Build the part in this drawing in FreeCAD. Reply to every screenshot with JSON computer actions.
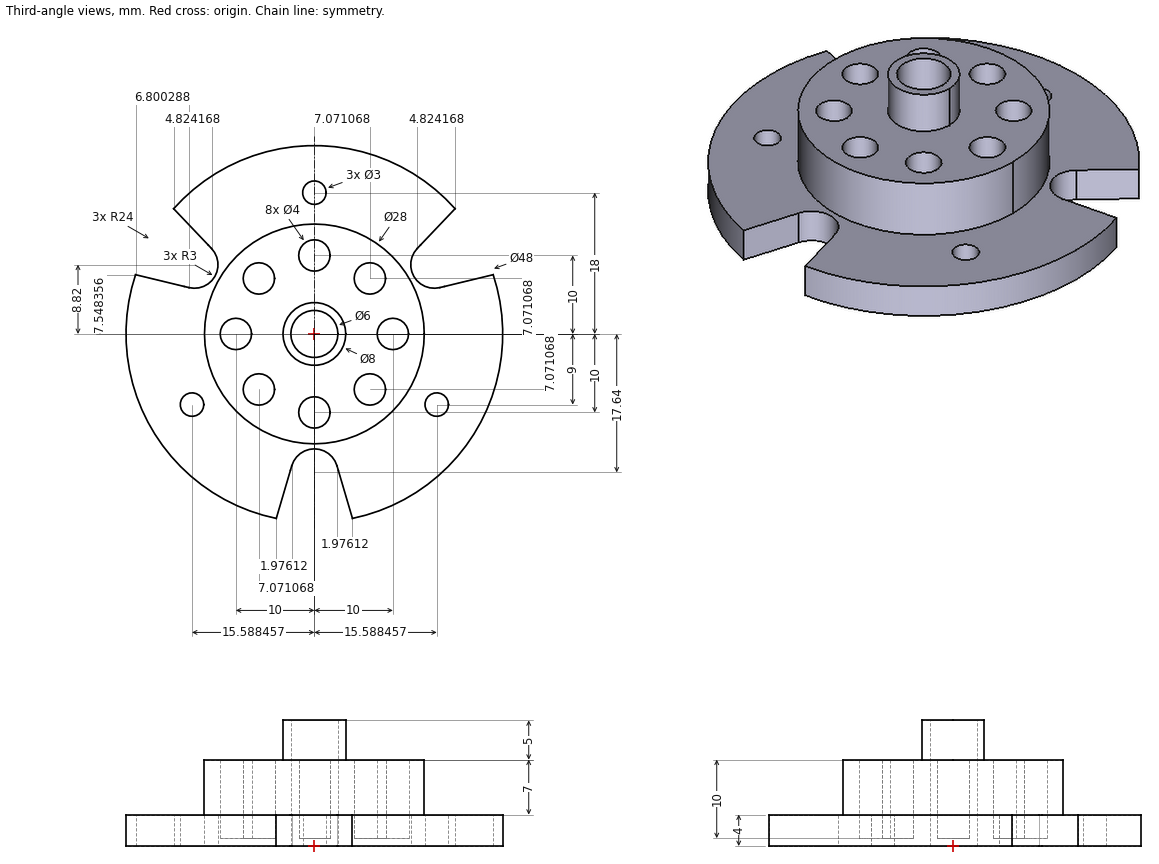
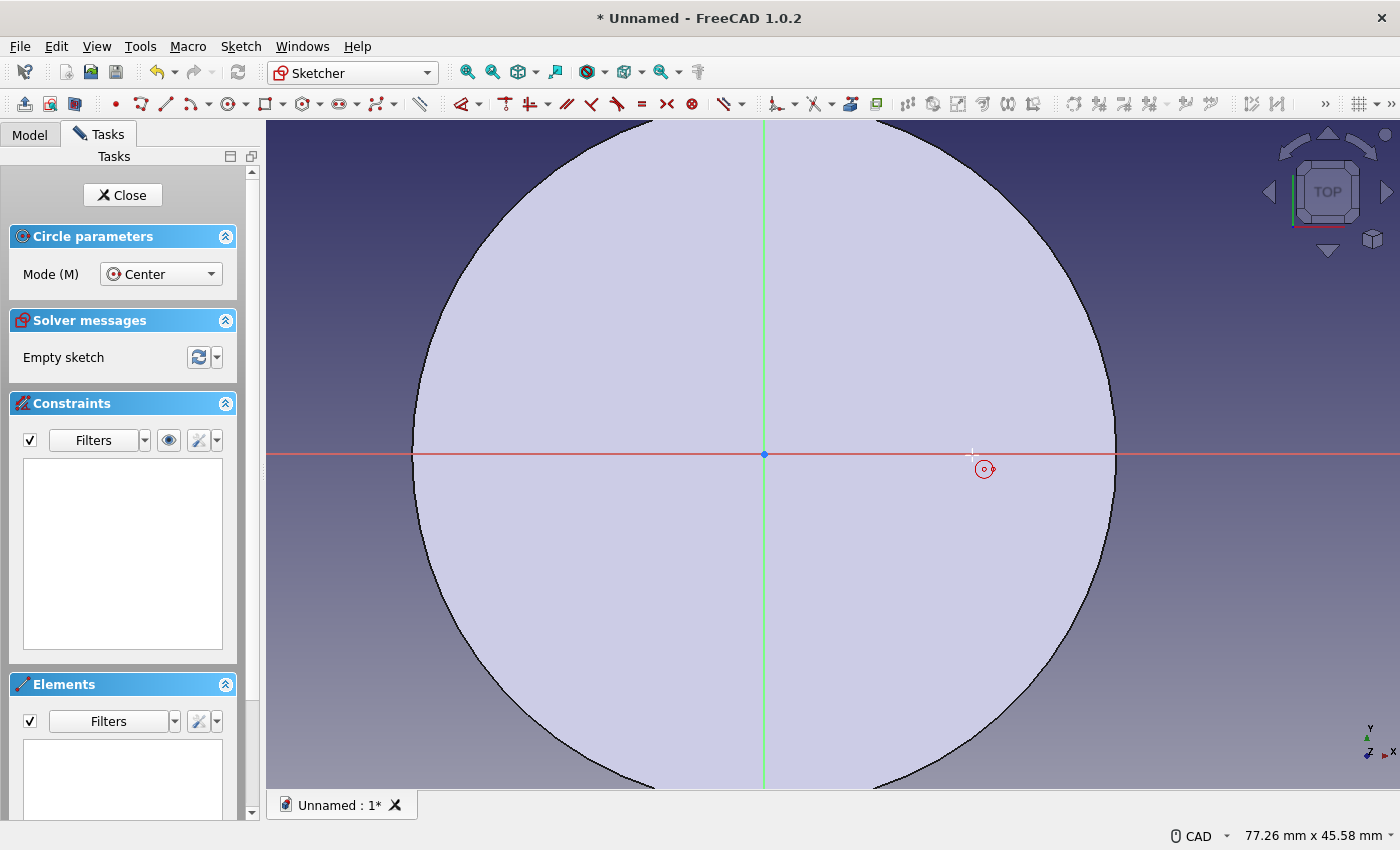
{"action": "left_click", "coordinate": [764, 454]}
{"action": "mouse_move", "coordinate": [910, 309]}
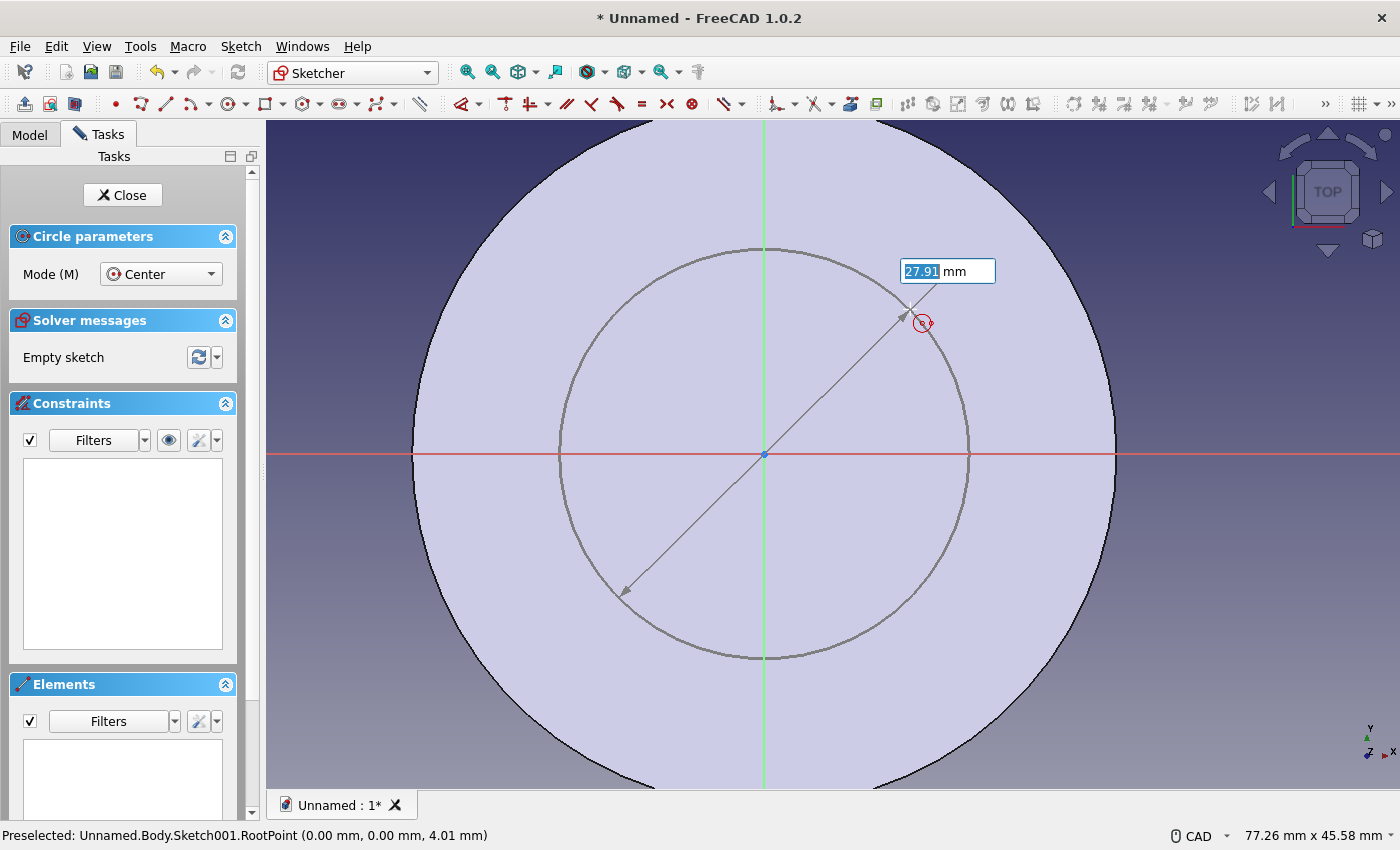
{"action": "type", "text": "28"}
{"action": "key", "text": "Return"}
{"action": "key", "text": "Escape"}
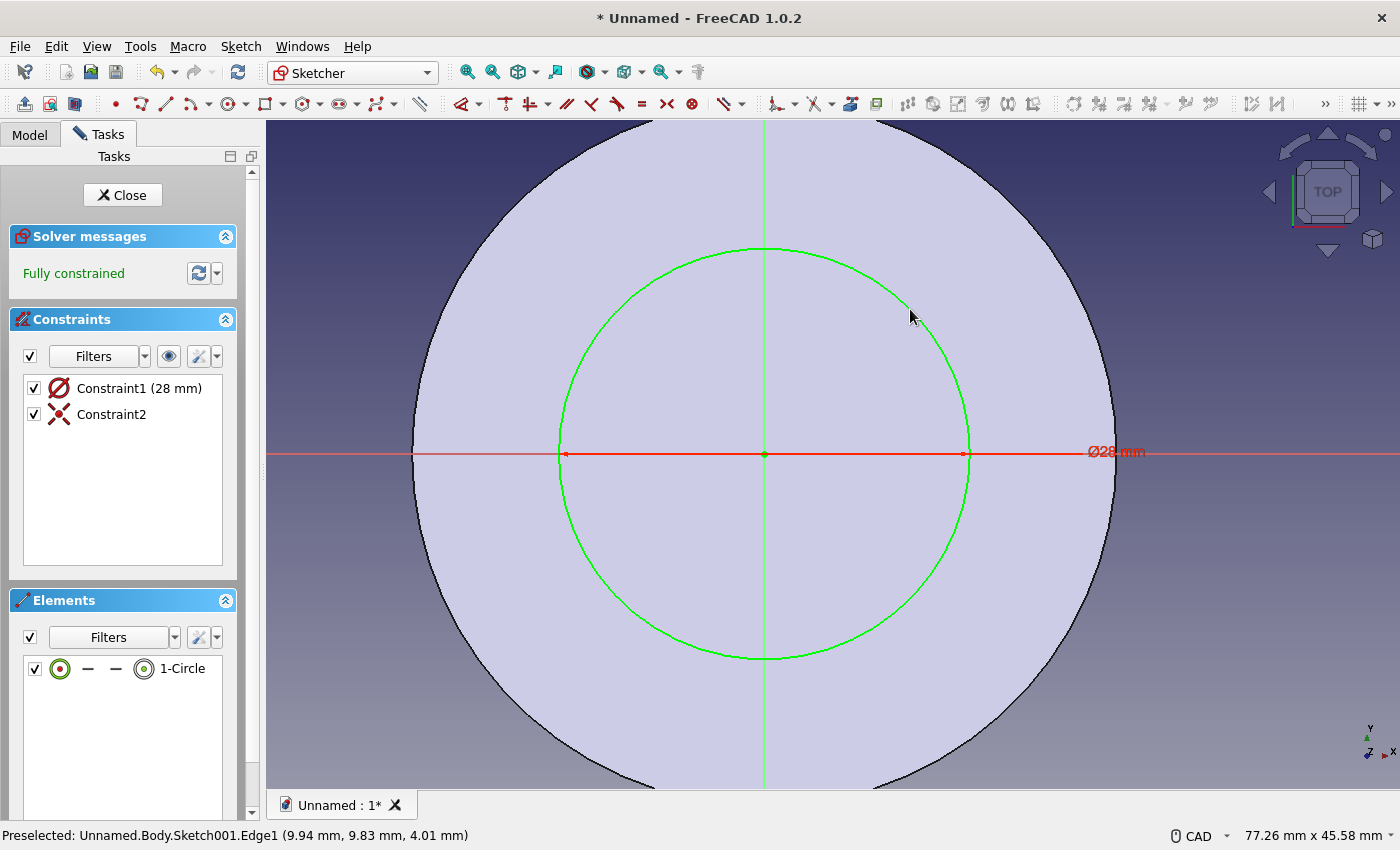
{"action": "left_click", "coordinate": [123, 195]}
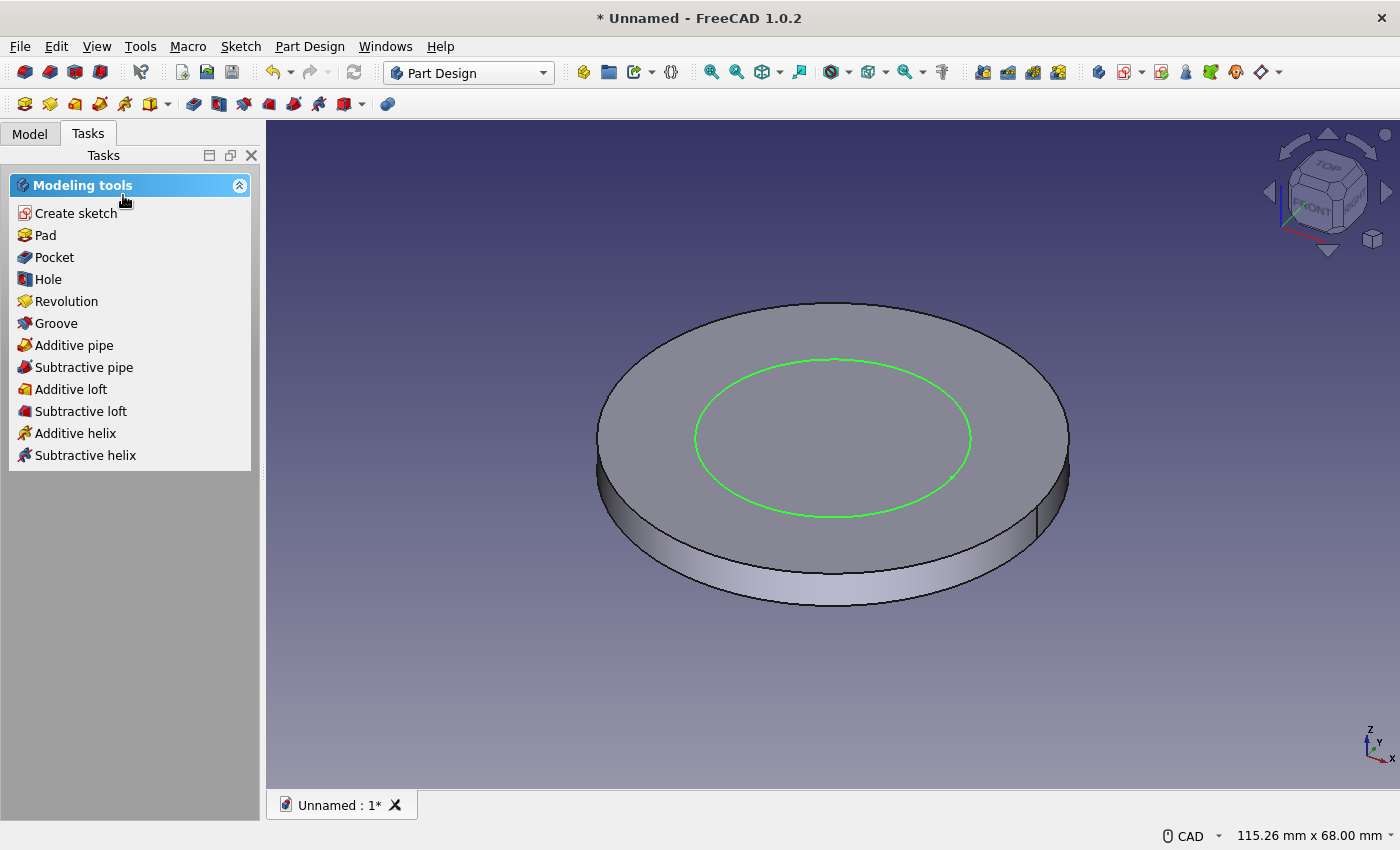
{"action": "left_click", "coordinate": [25, 104]}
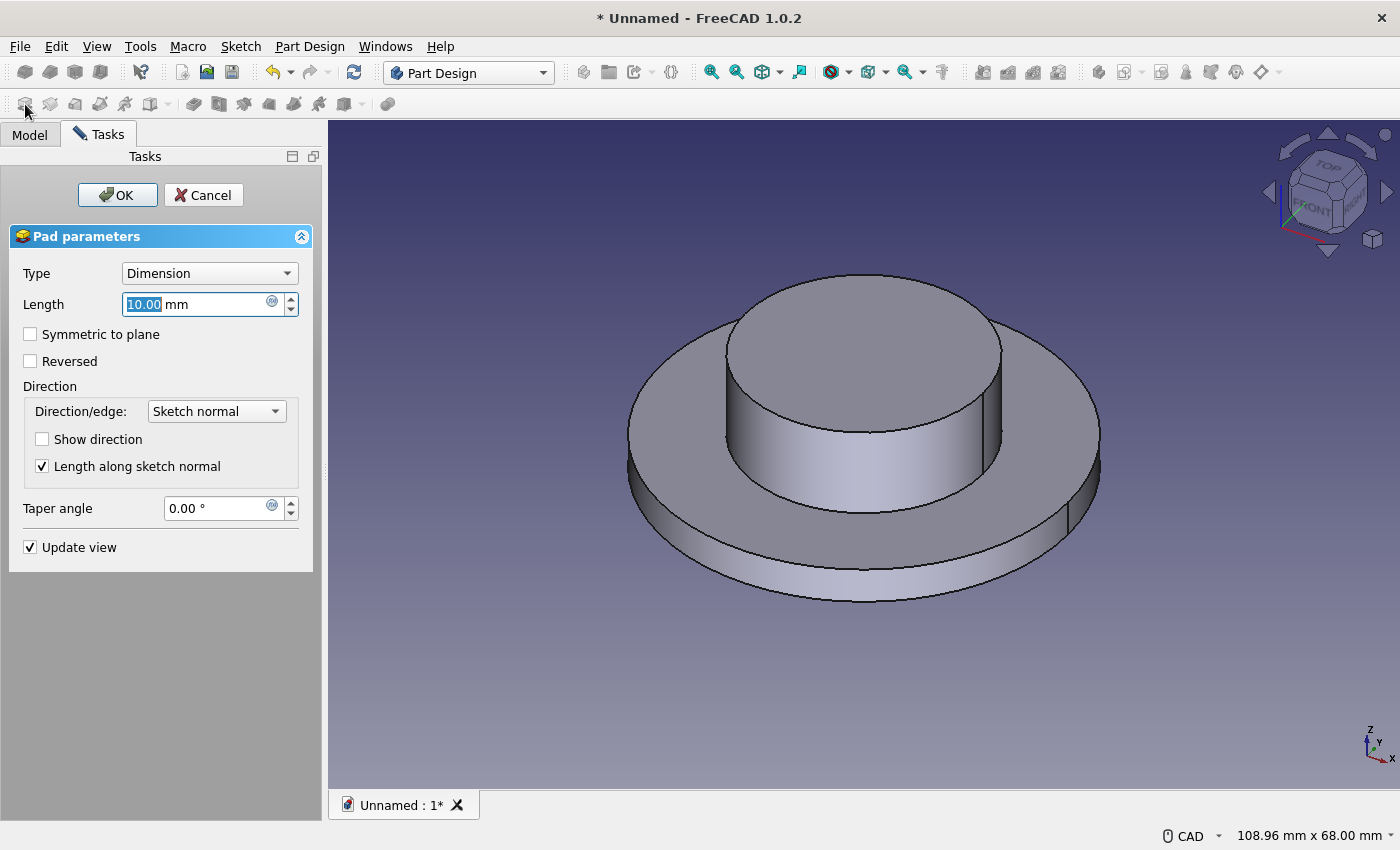
{"action": "type", "text": "7"}
{"action": "key", "text": "Tab"}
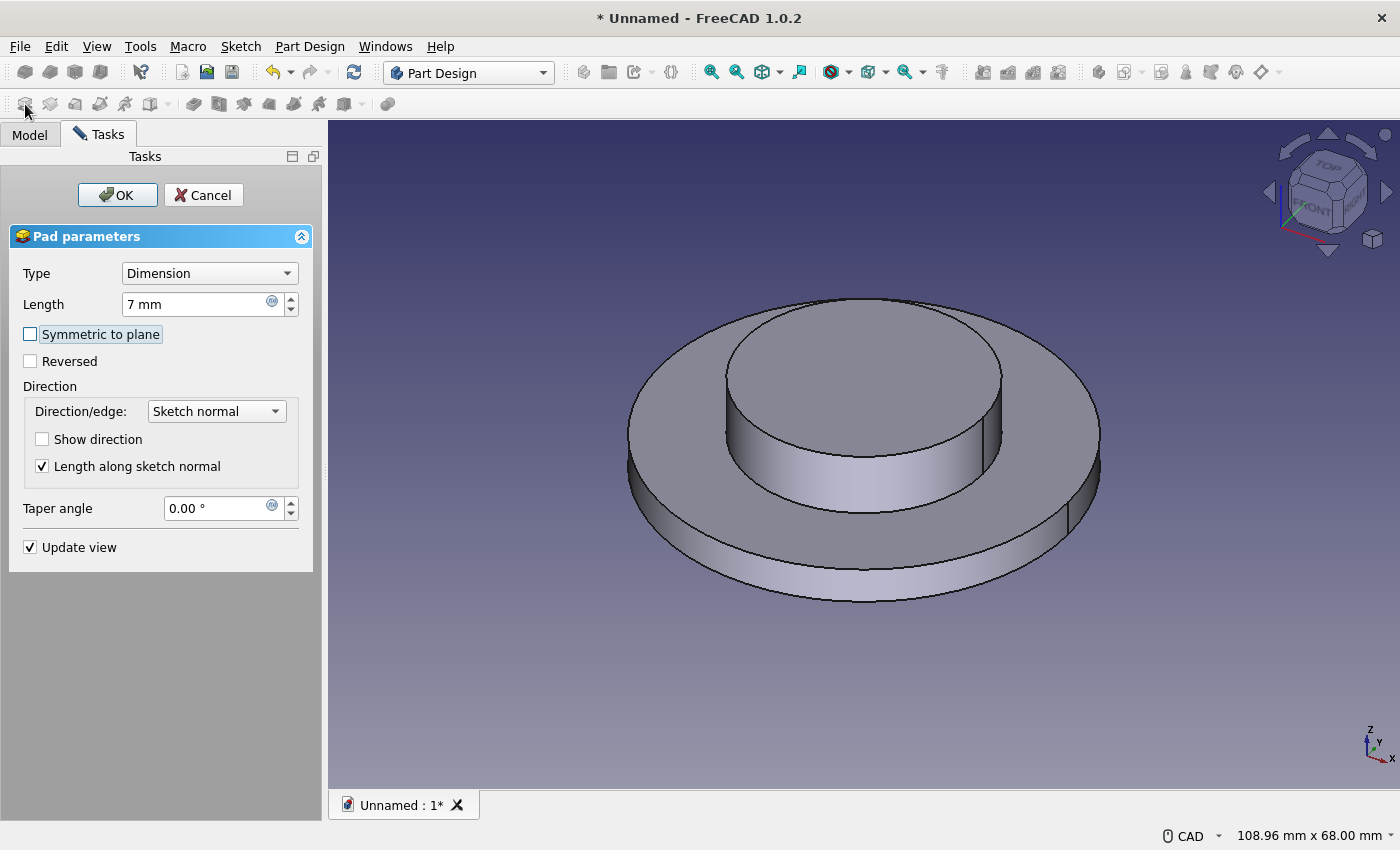
{"action": "left_click", "coordinate": [118, 195]}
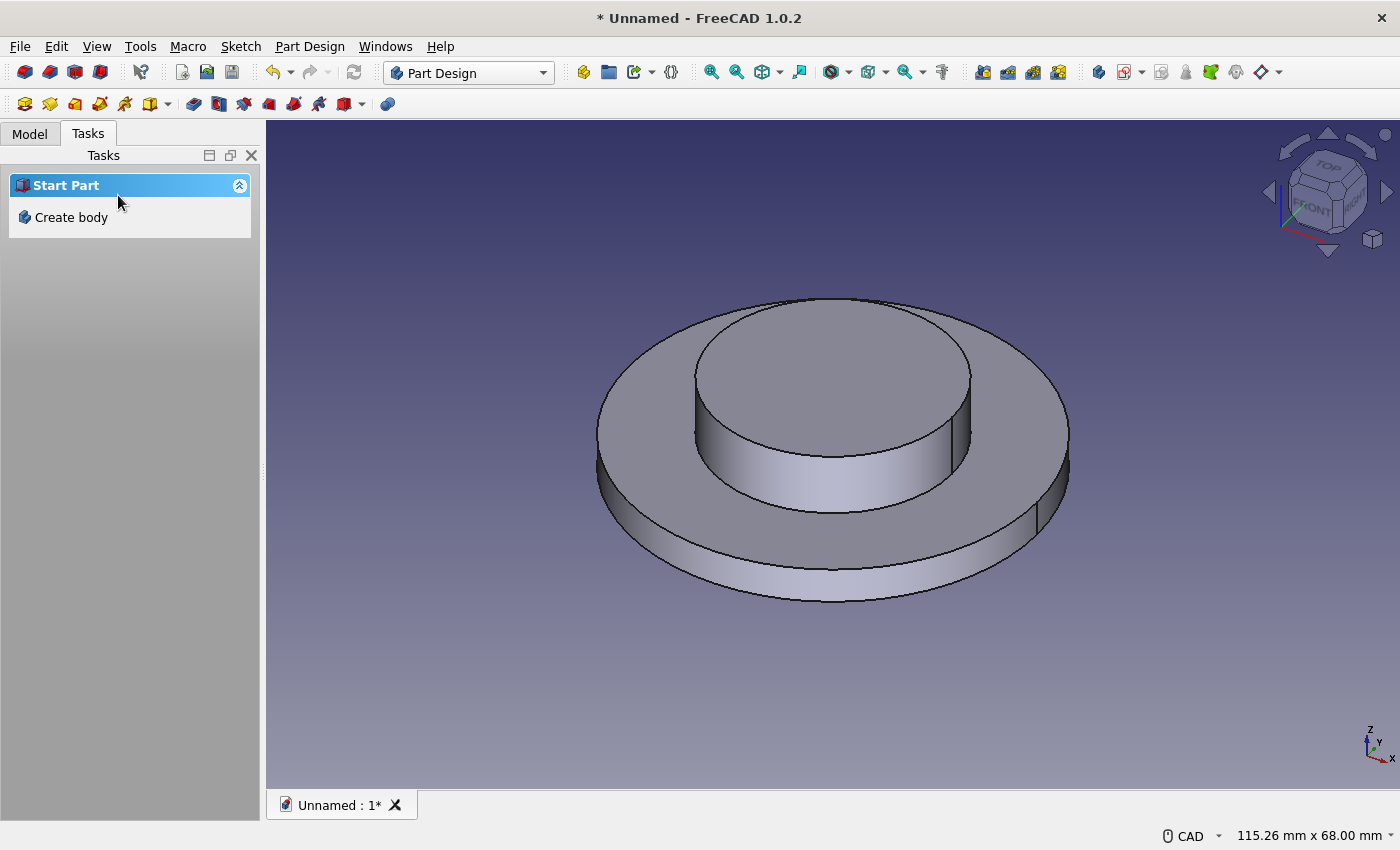
{"action": "left_click", "coordinate": [1017, 405]}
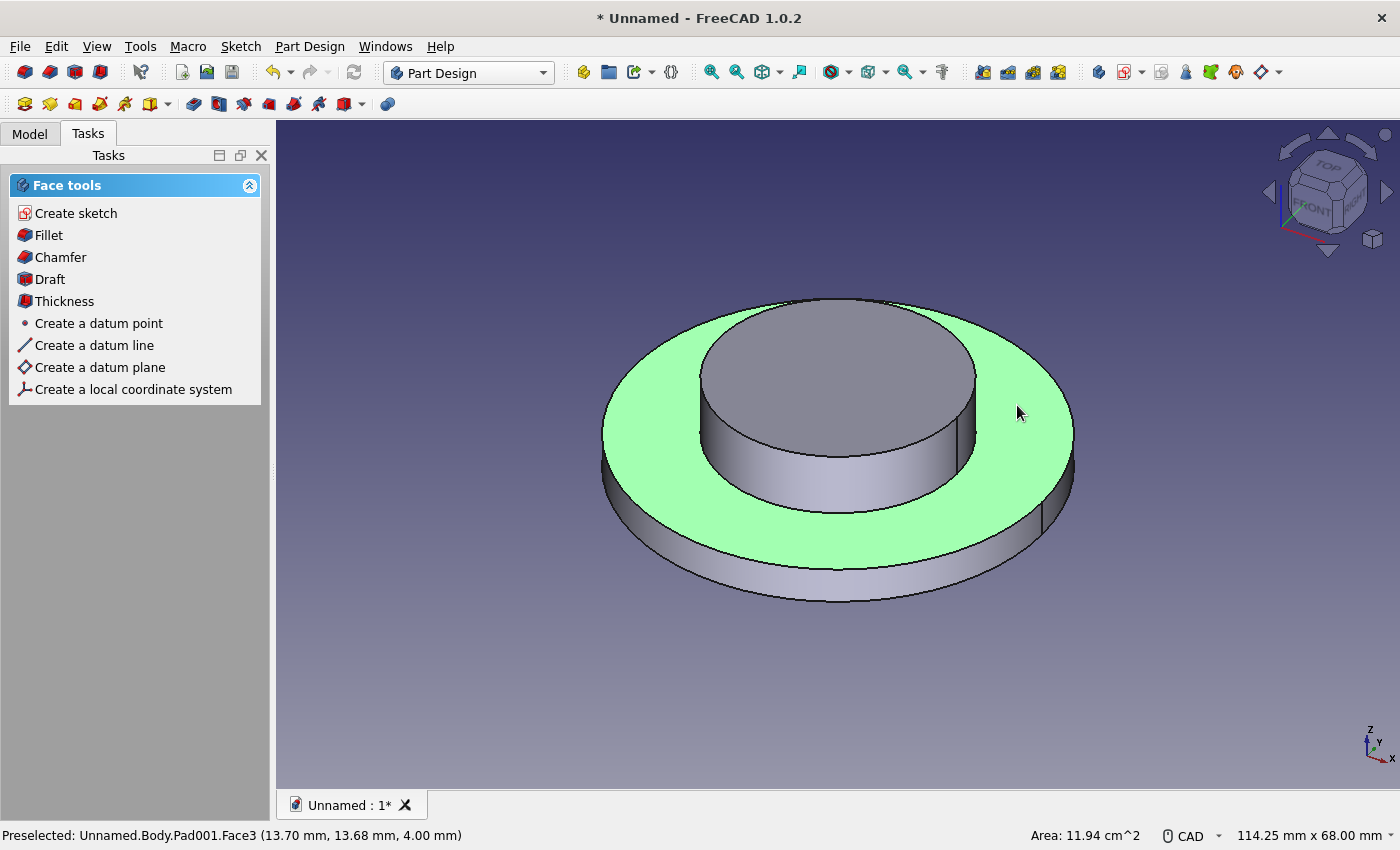
{"action": "left_click", "coordinate": [1124, 72]}